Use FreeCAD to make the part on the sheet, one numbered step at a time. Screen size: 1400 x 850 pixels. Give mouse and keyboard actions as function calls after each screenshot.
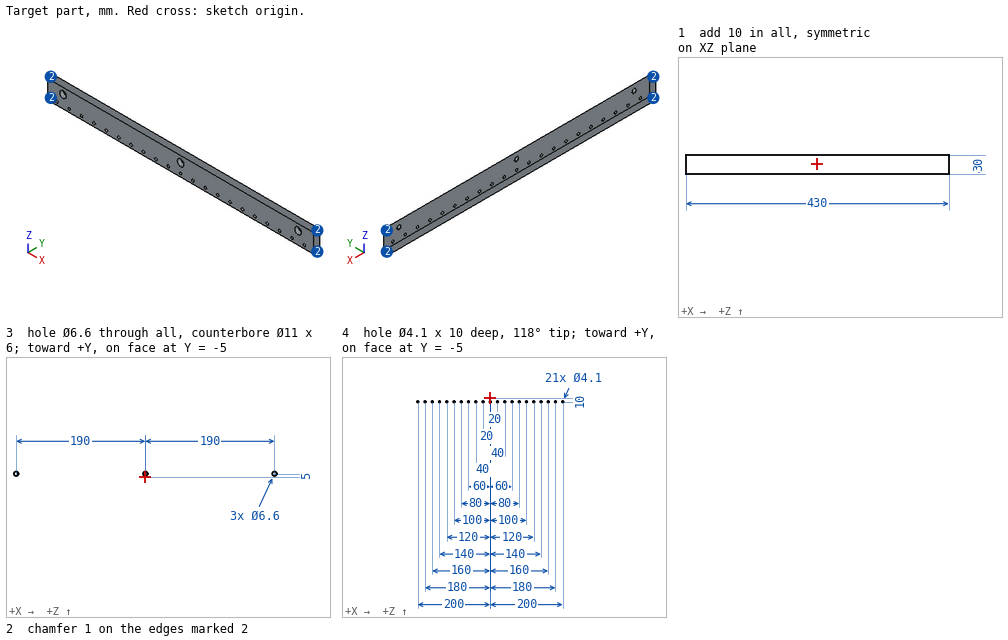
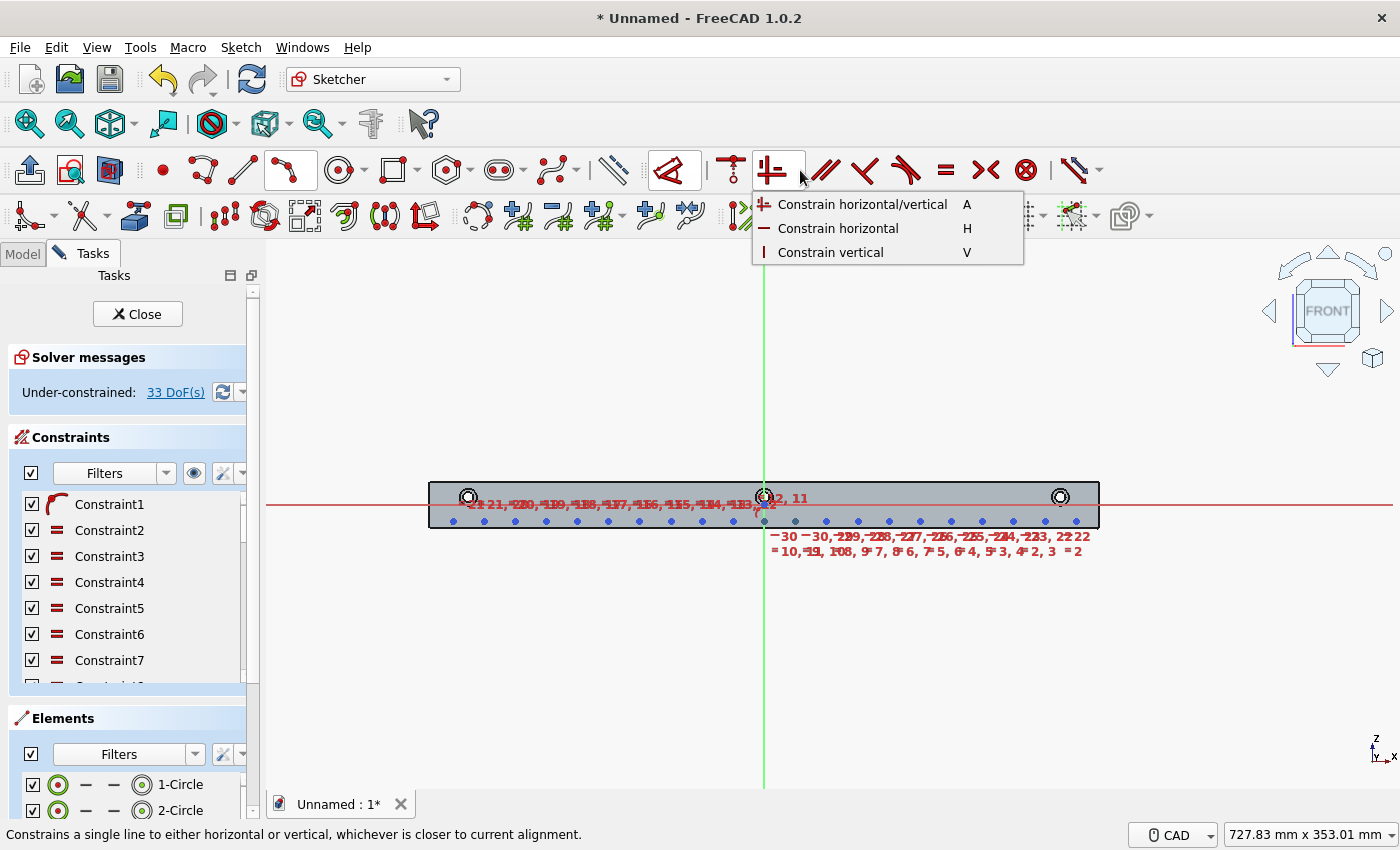
click(888, 228)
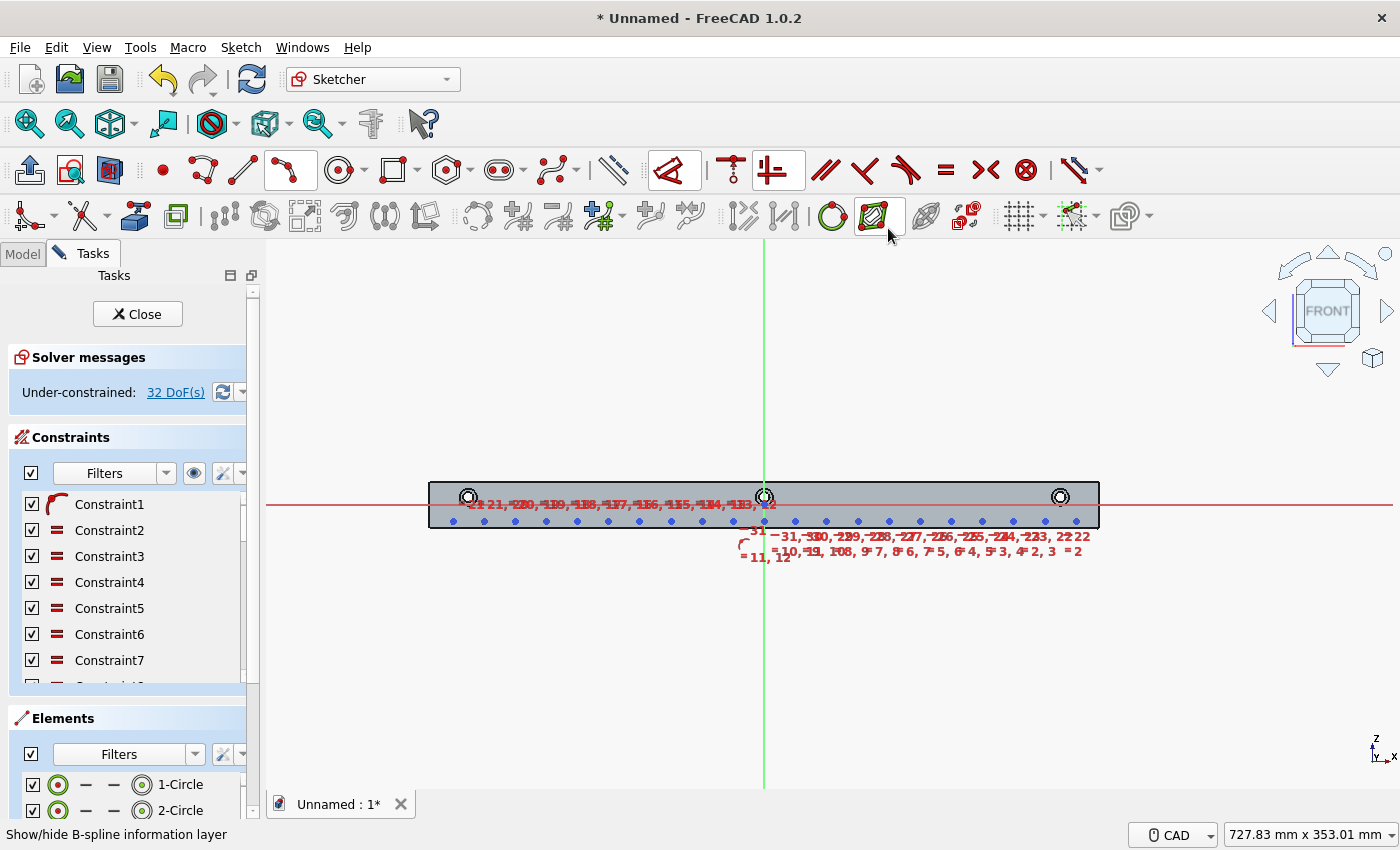
click(762, 520)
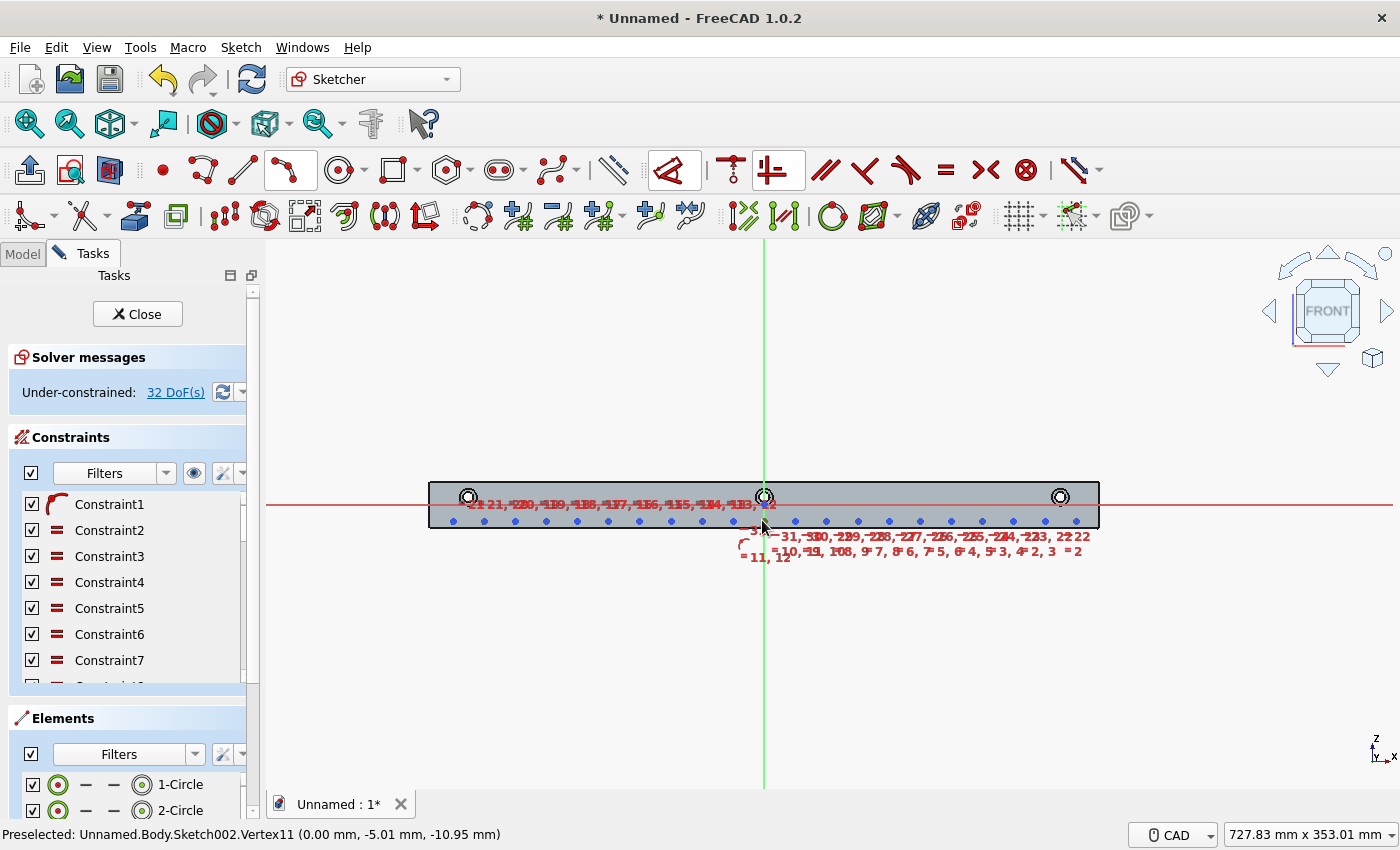
click(733, 522)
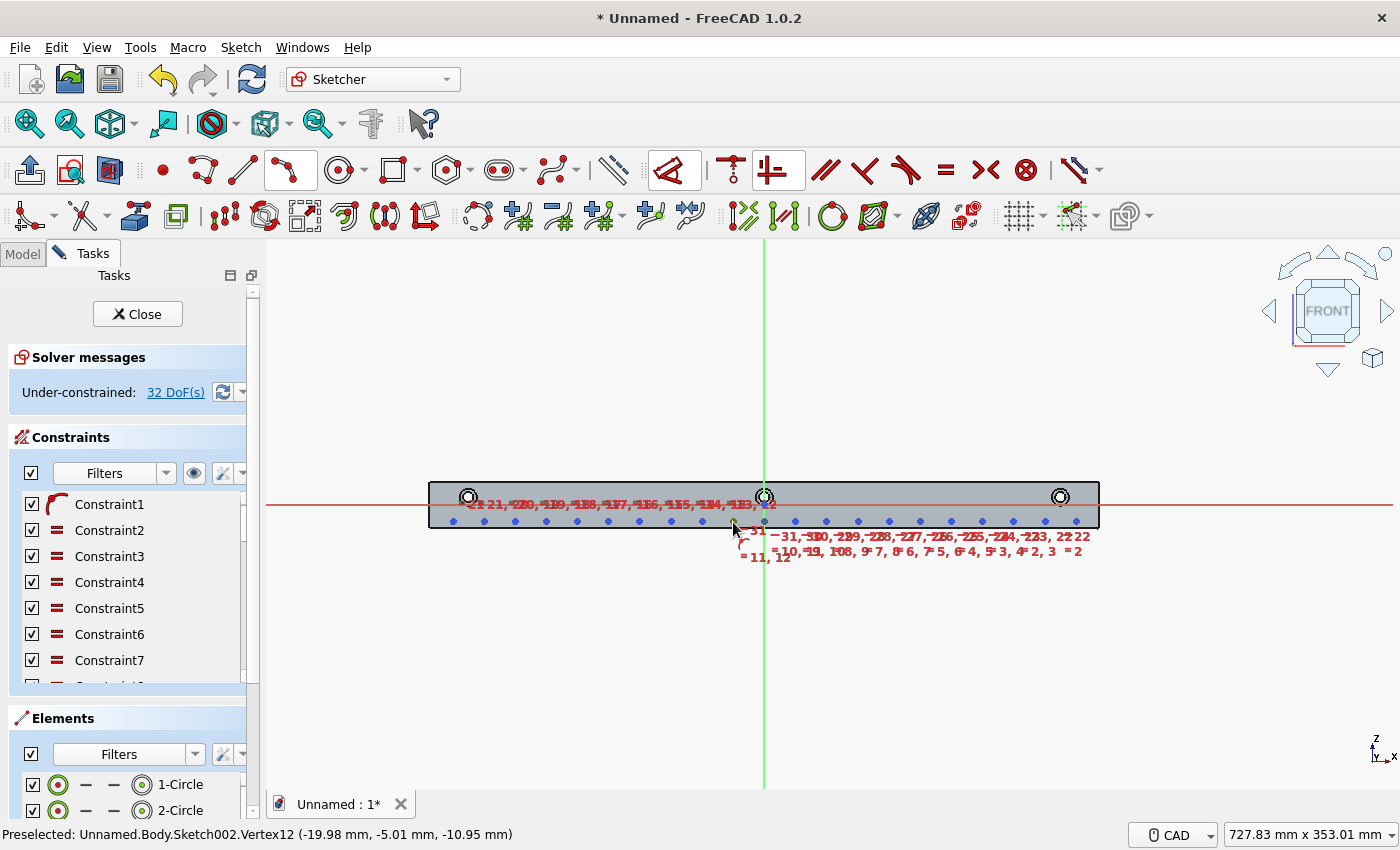
key(h)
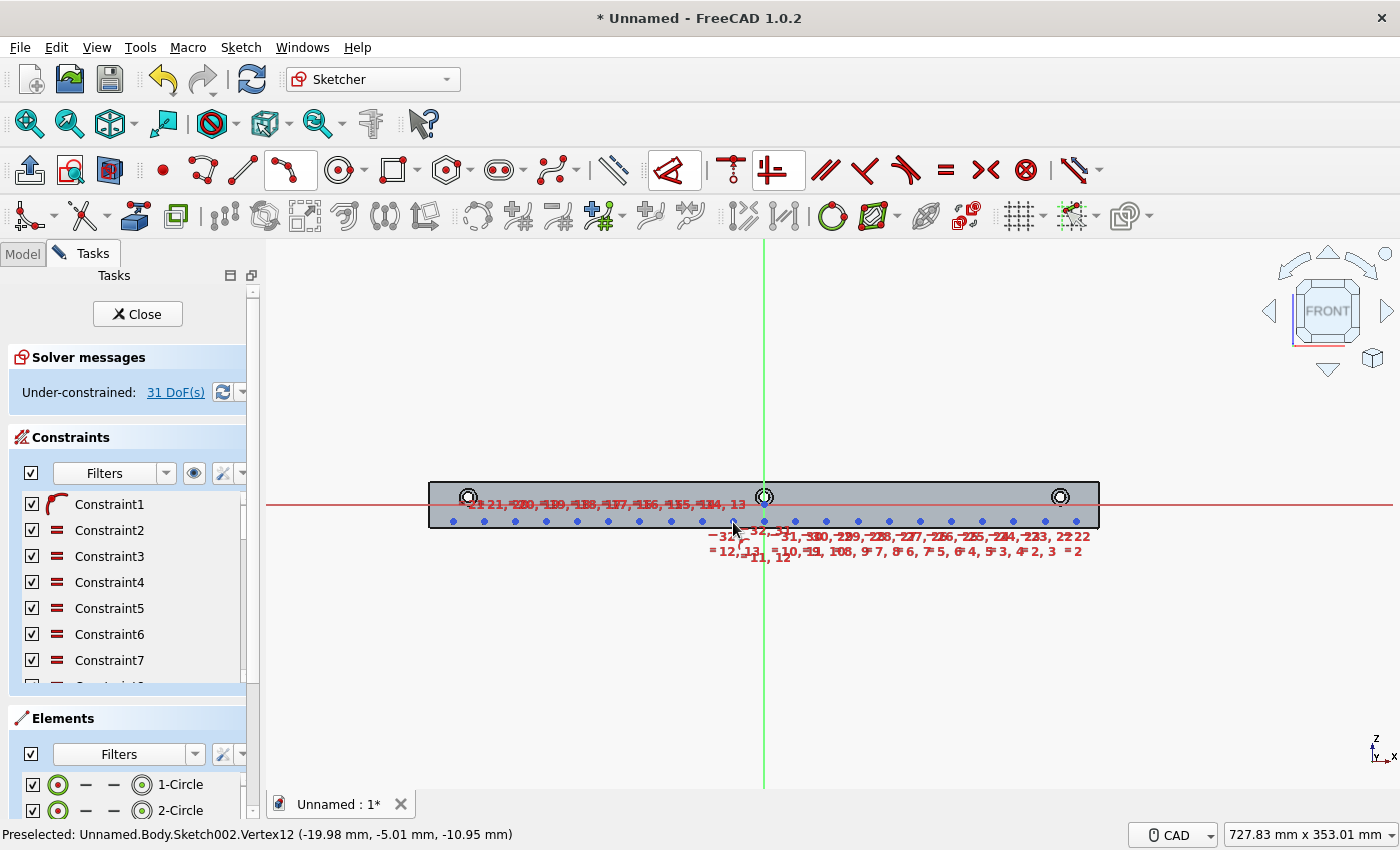
click(733, 522)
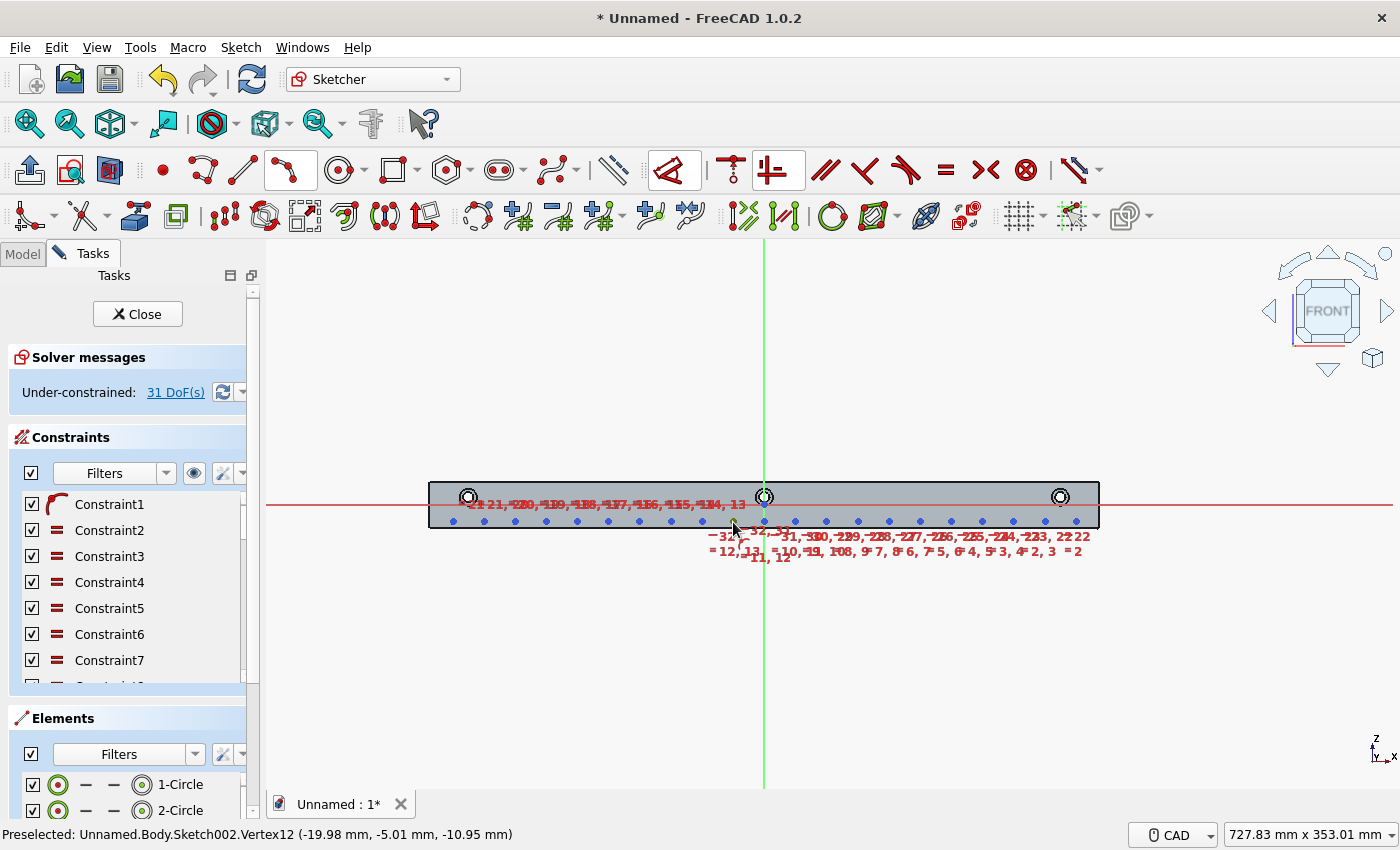
click(702, 522)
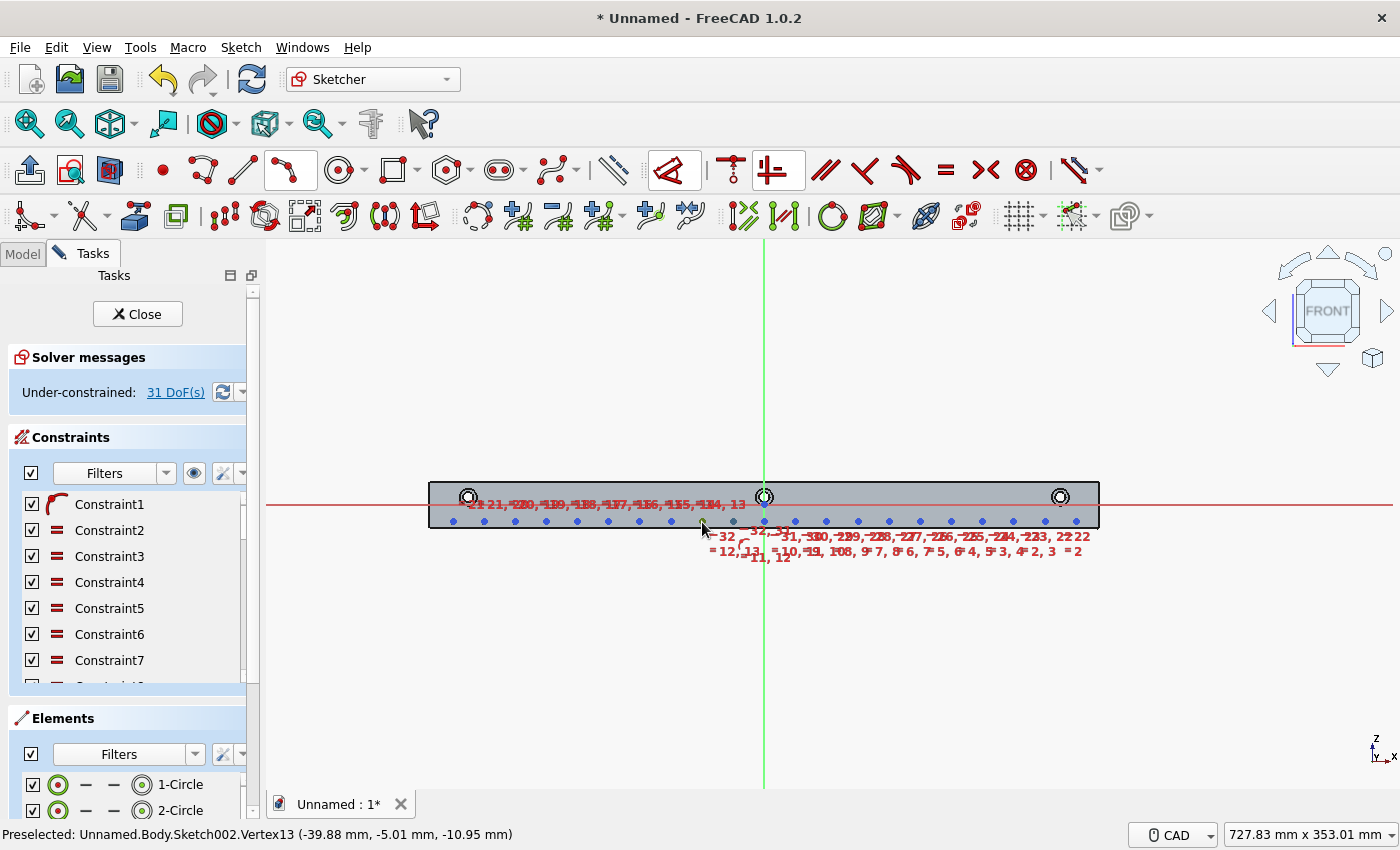
key(h)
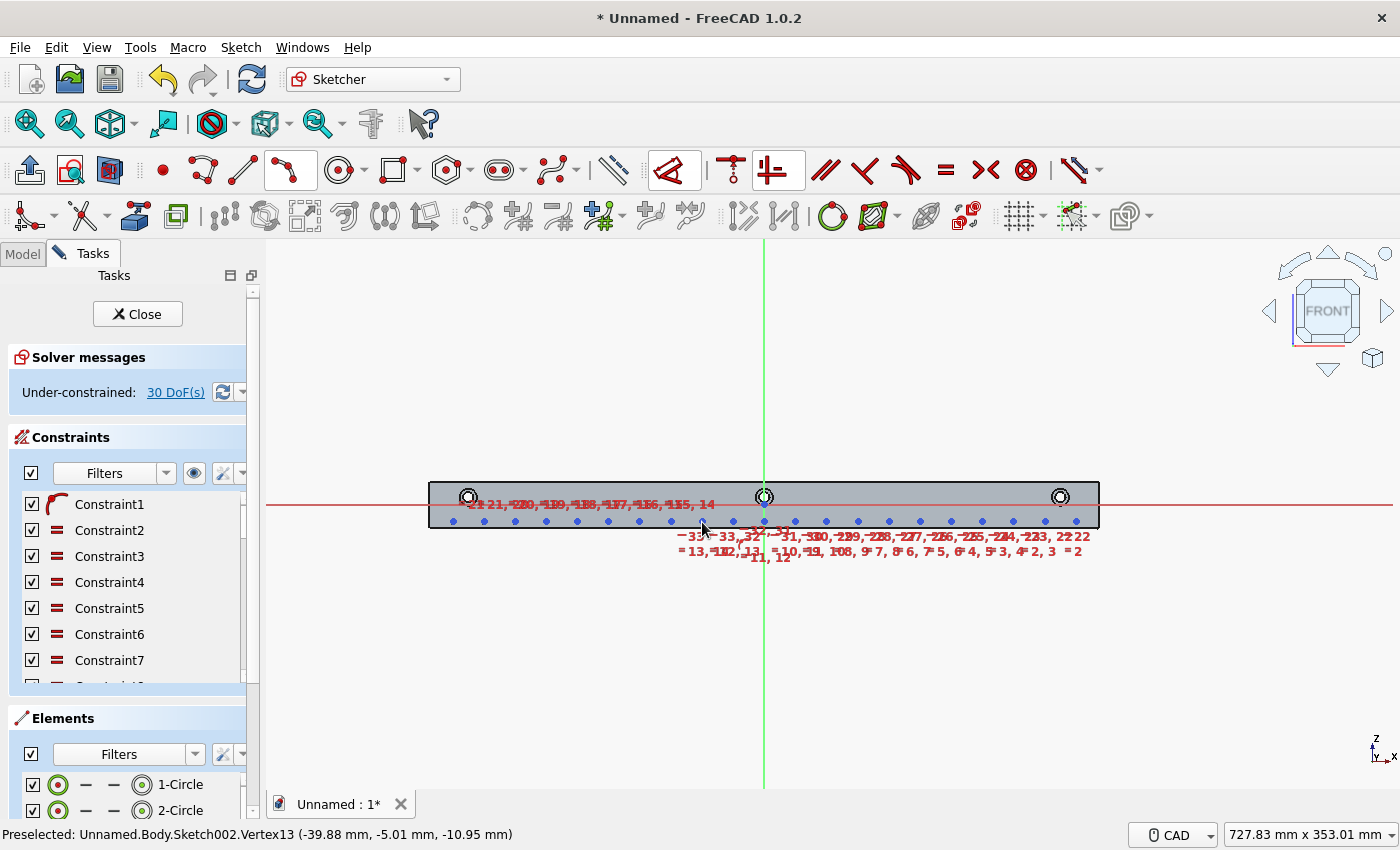
click(702, 522)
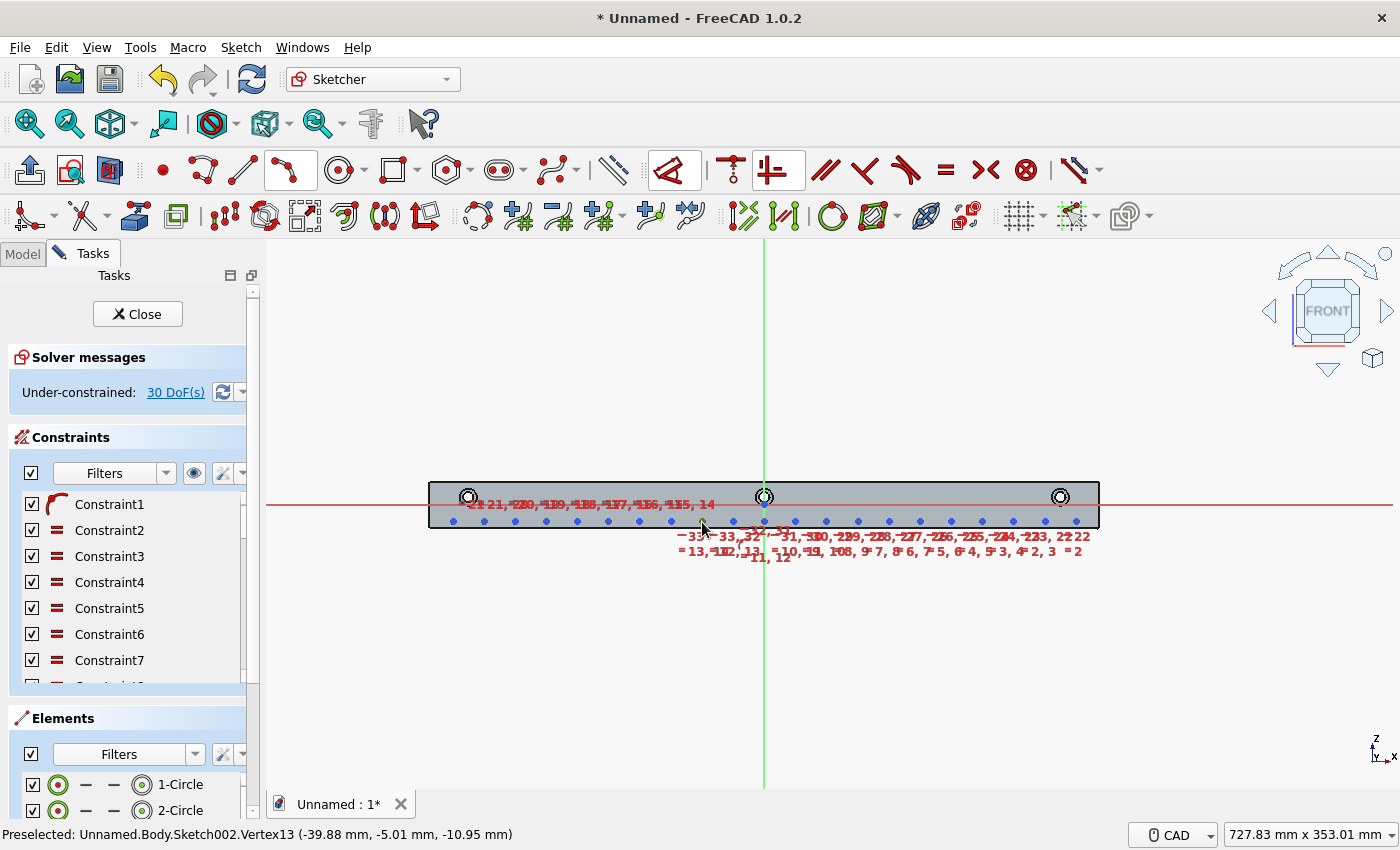
click(671, 522)